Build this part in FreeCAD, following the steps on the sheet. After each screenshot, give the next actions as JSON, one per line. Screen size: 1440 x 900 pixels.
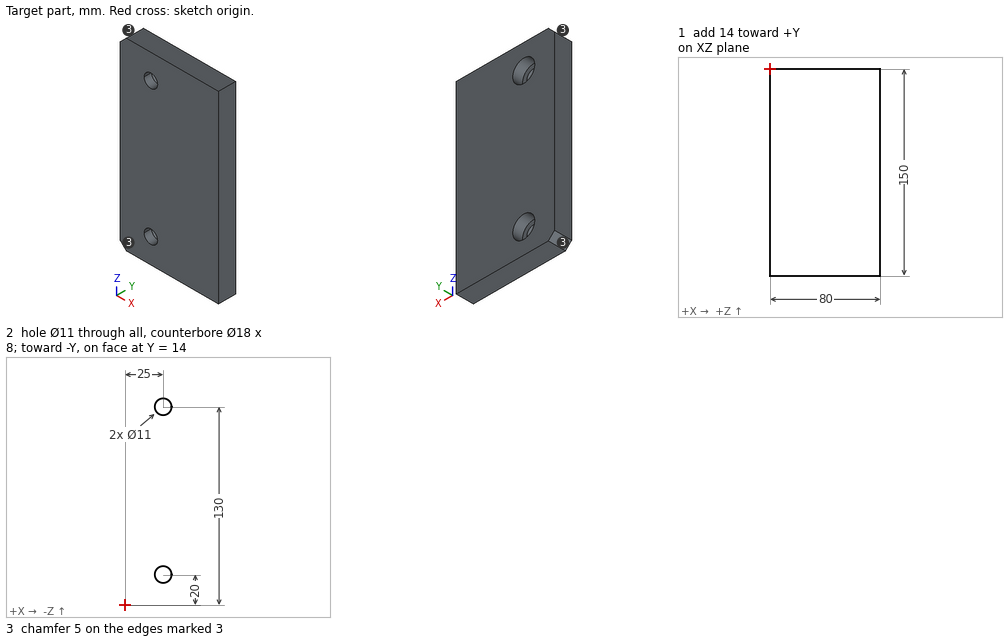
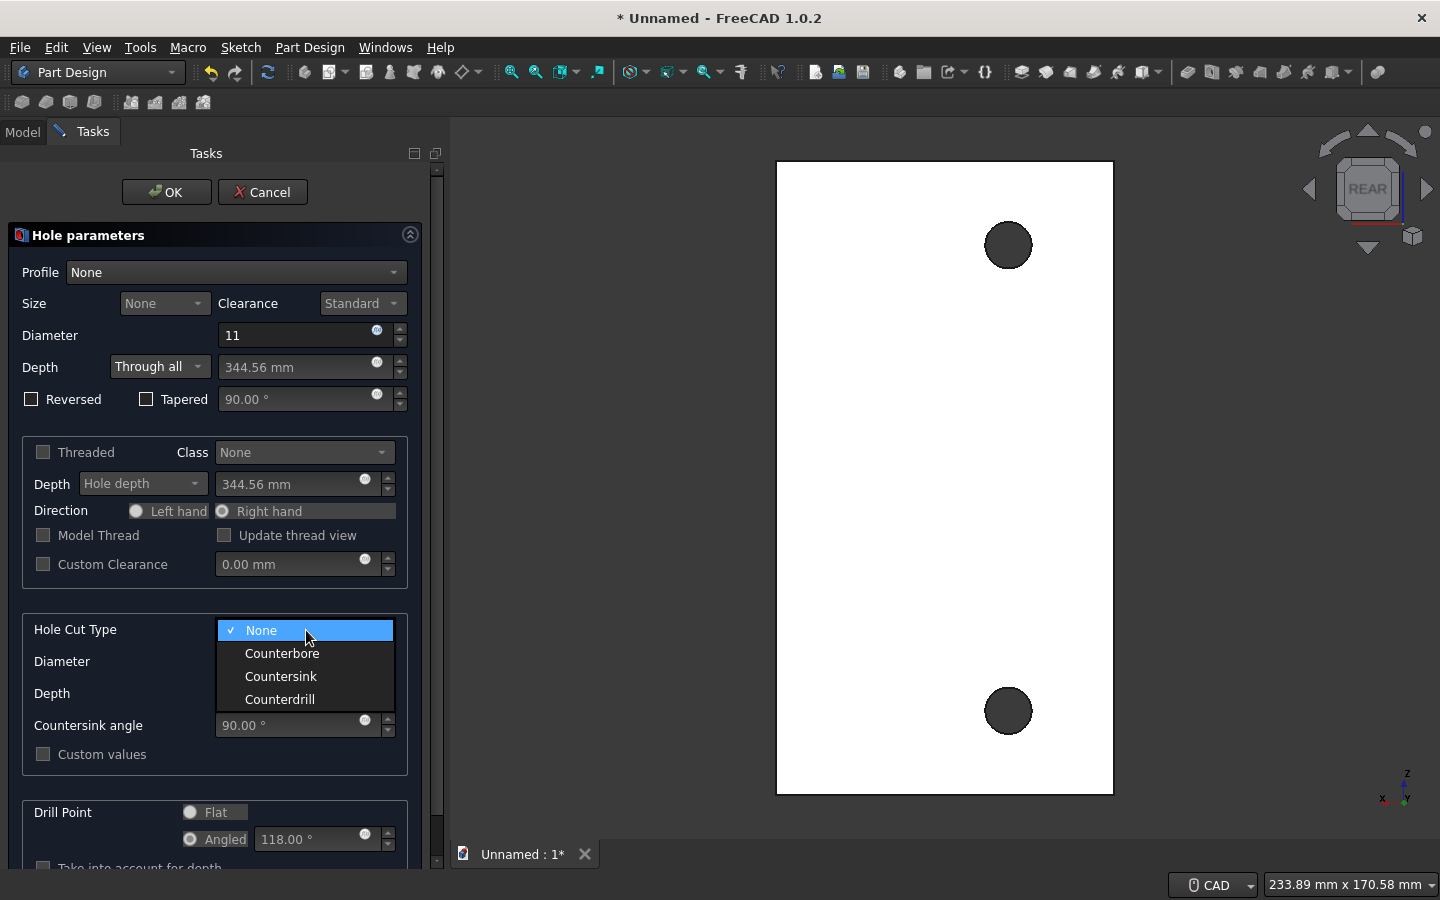
{"action": "left_click", "coordinate": [304, 654]}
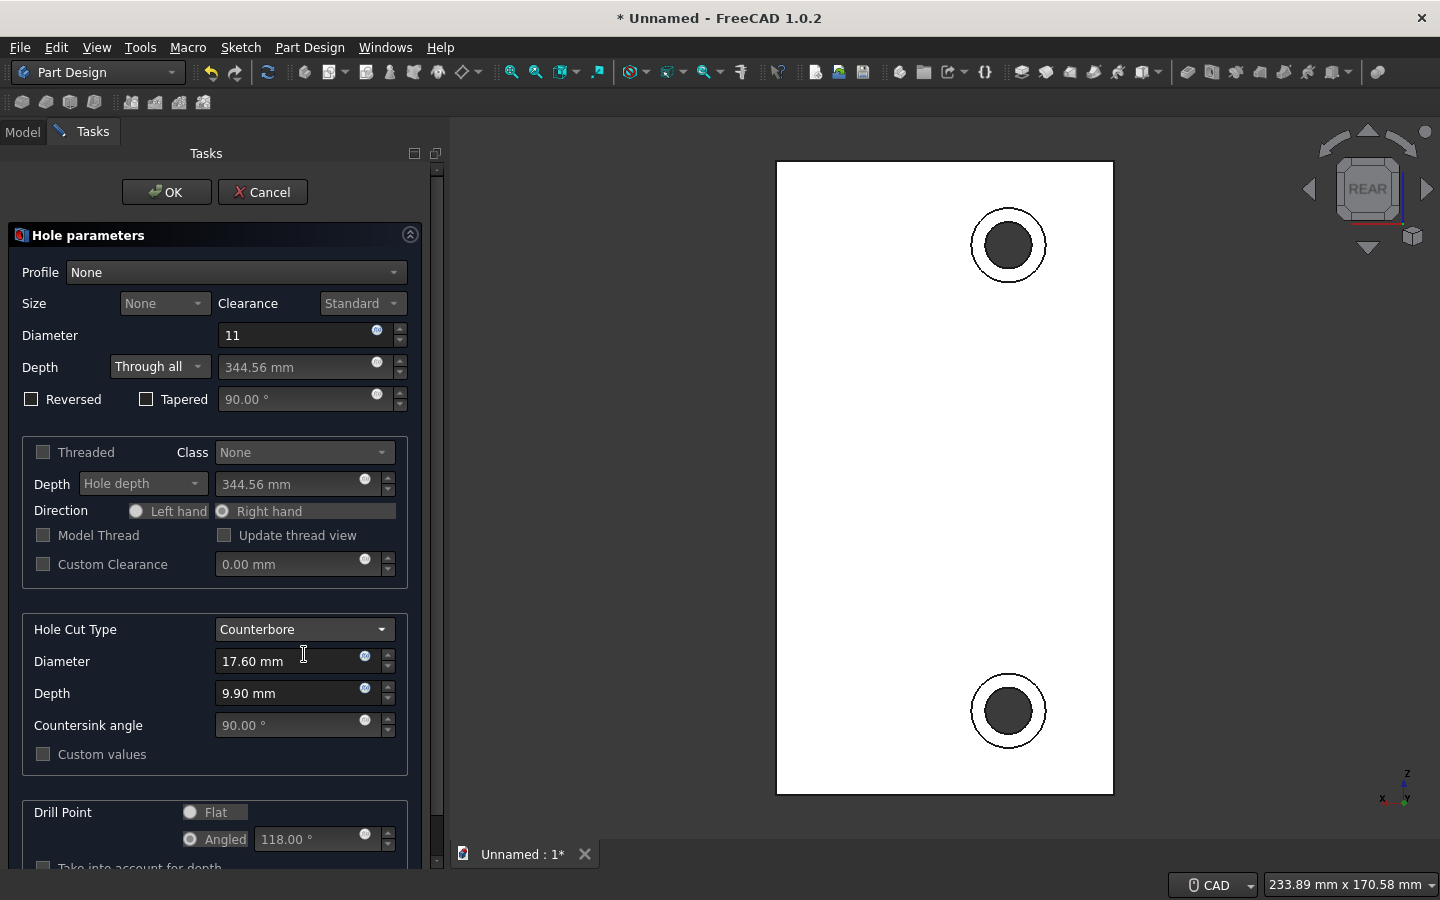
{"action": "triple_click", "coordinate": [298, 661]}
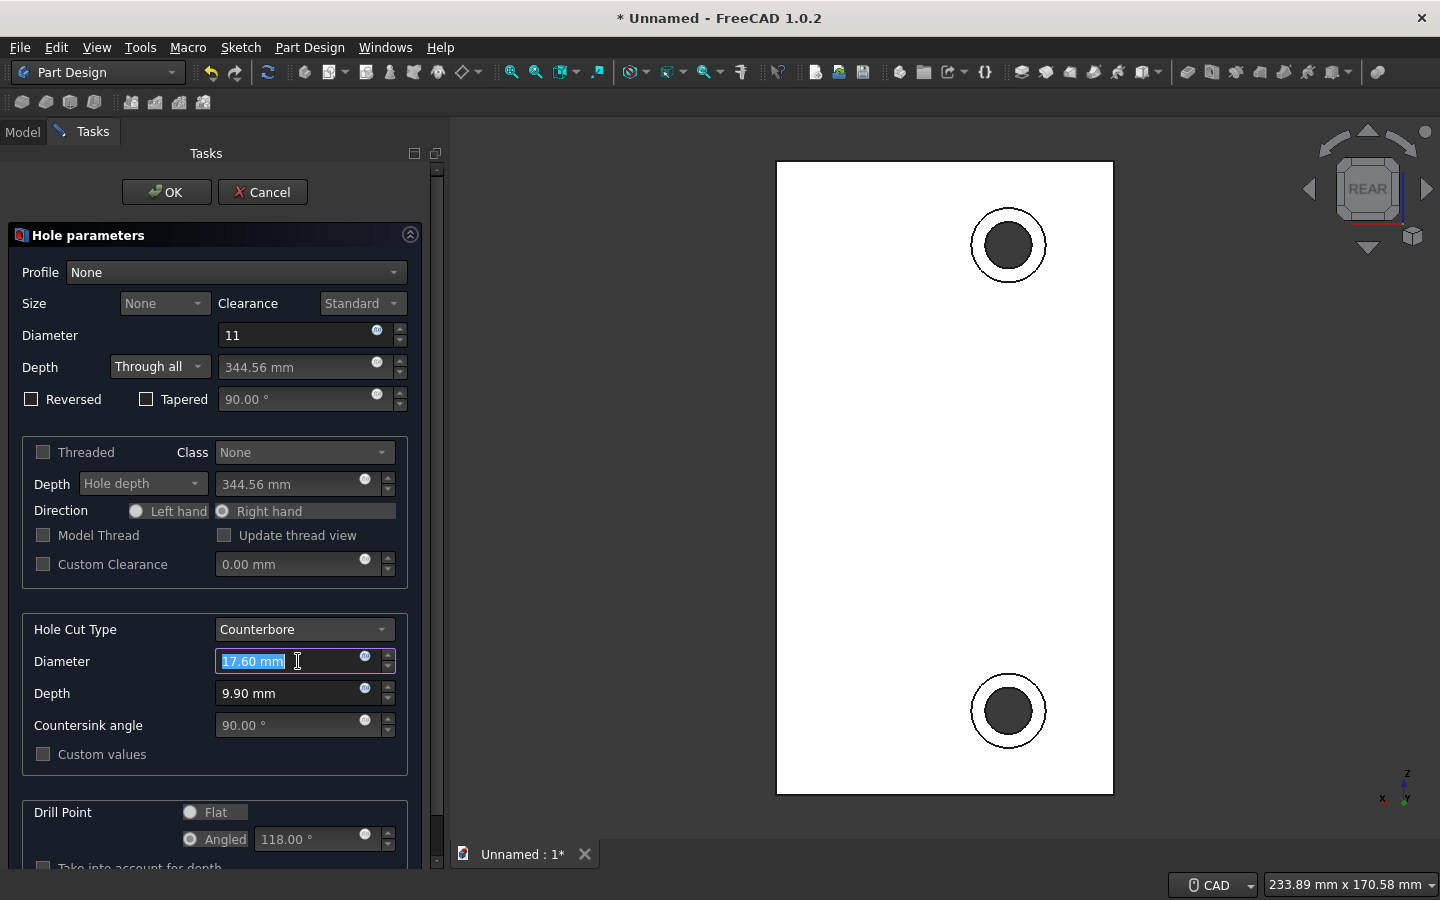
{"action": "type", "text": "18"}
{"action": "key", "text": "Tab"}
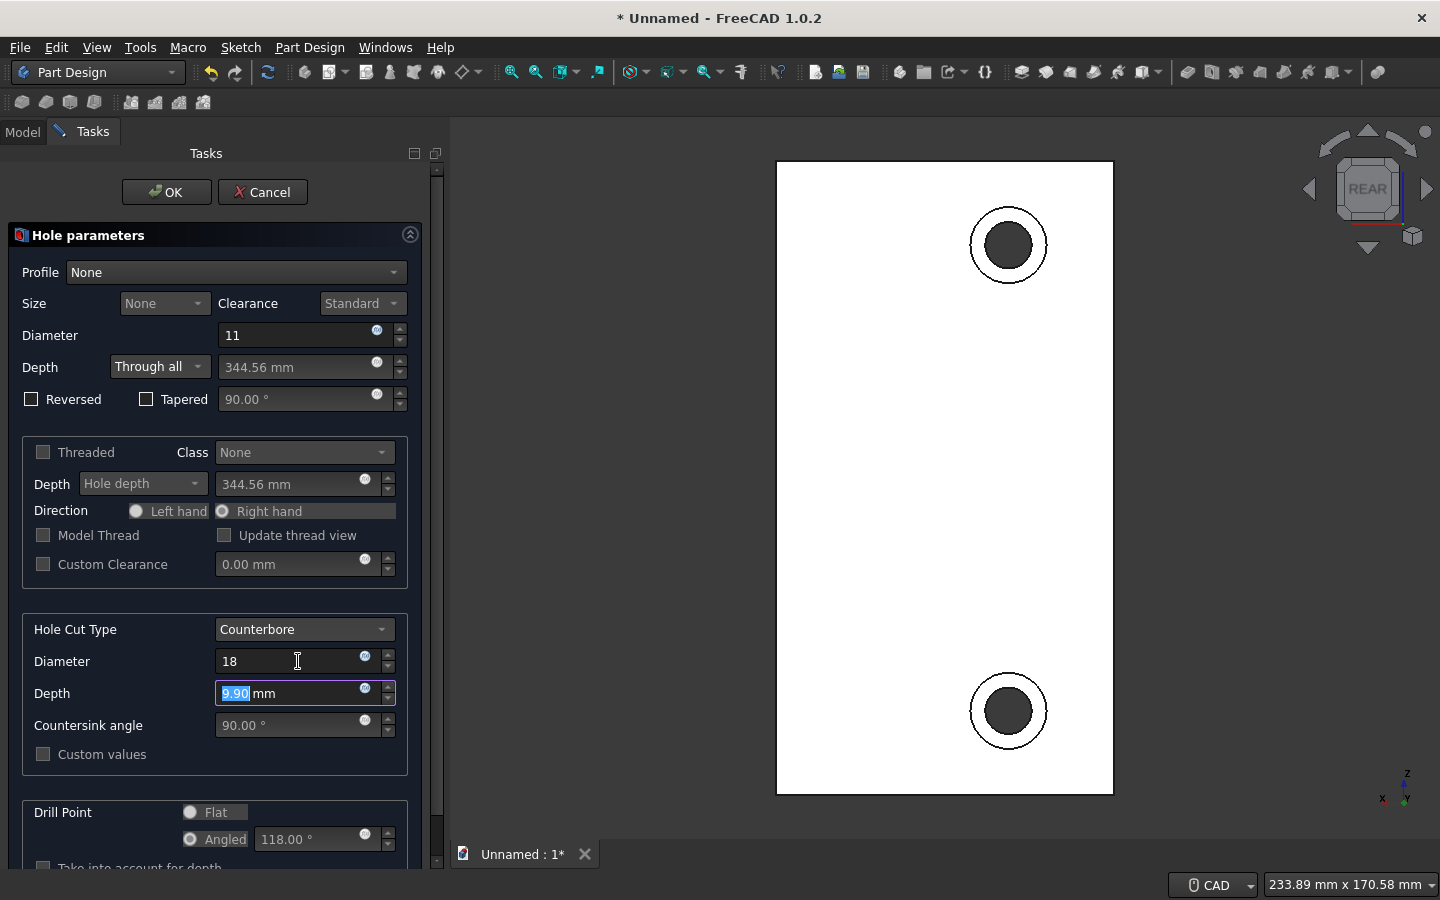
{"action": "type", "text": "8"}
{"action": "key", "text": "Tab"}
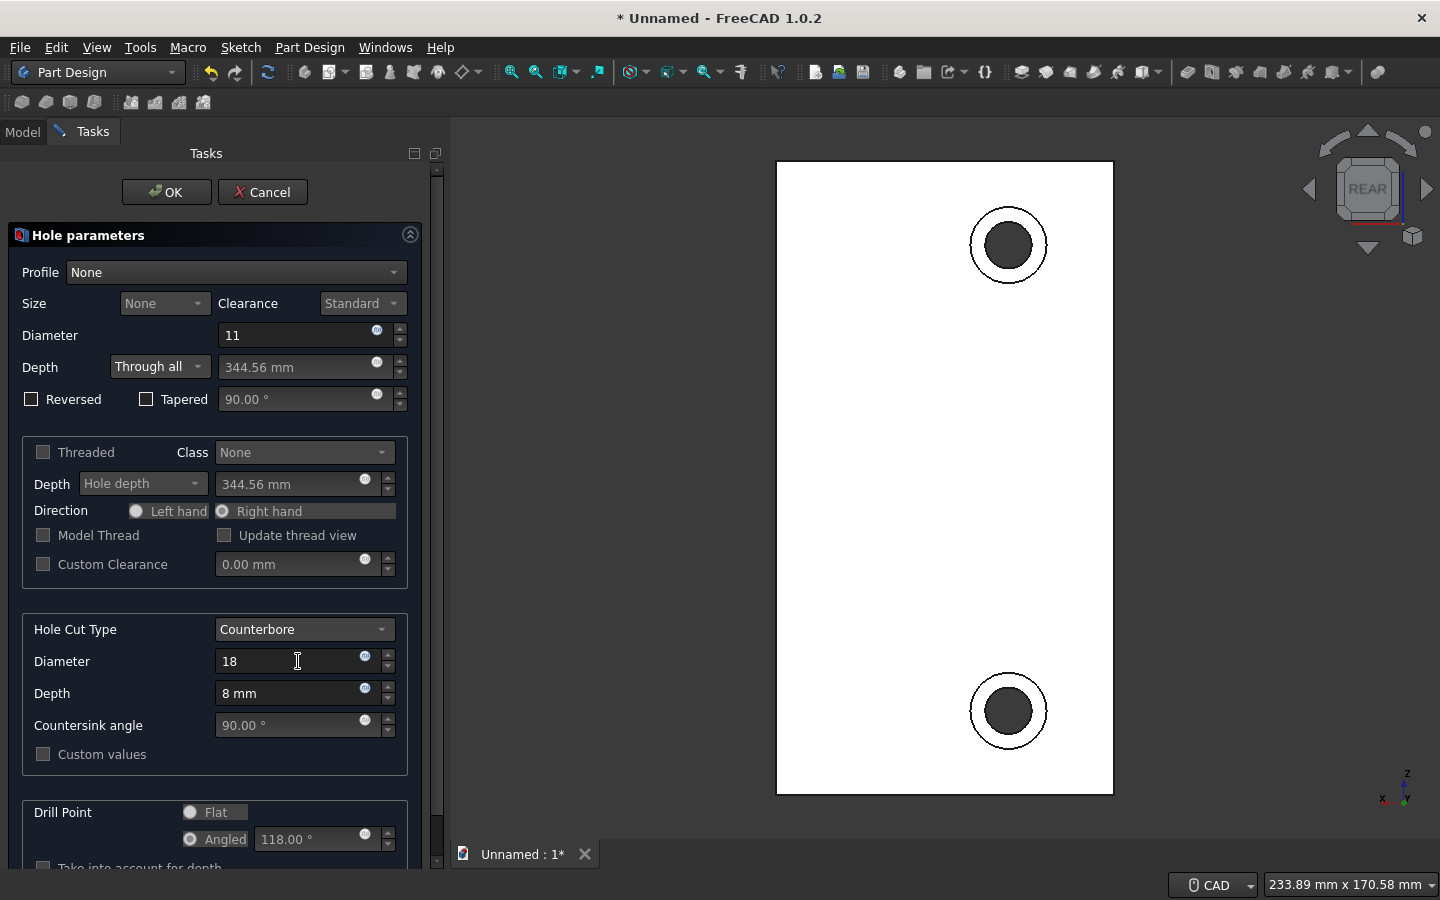
{"action": "left_click", "coordinate": [167, 192]}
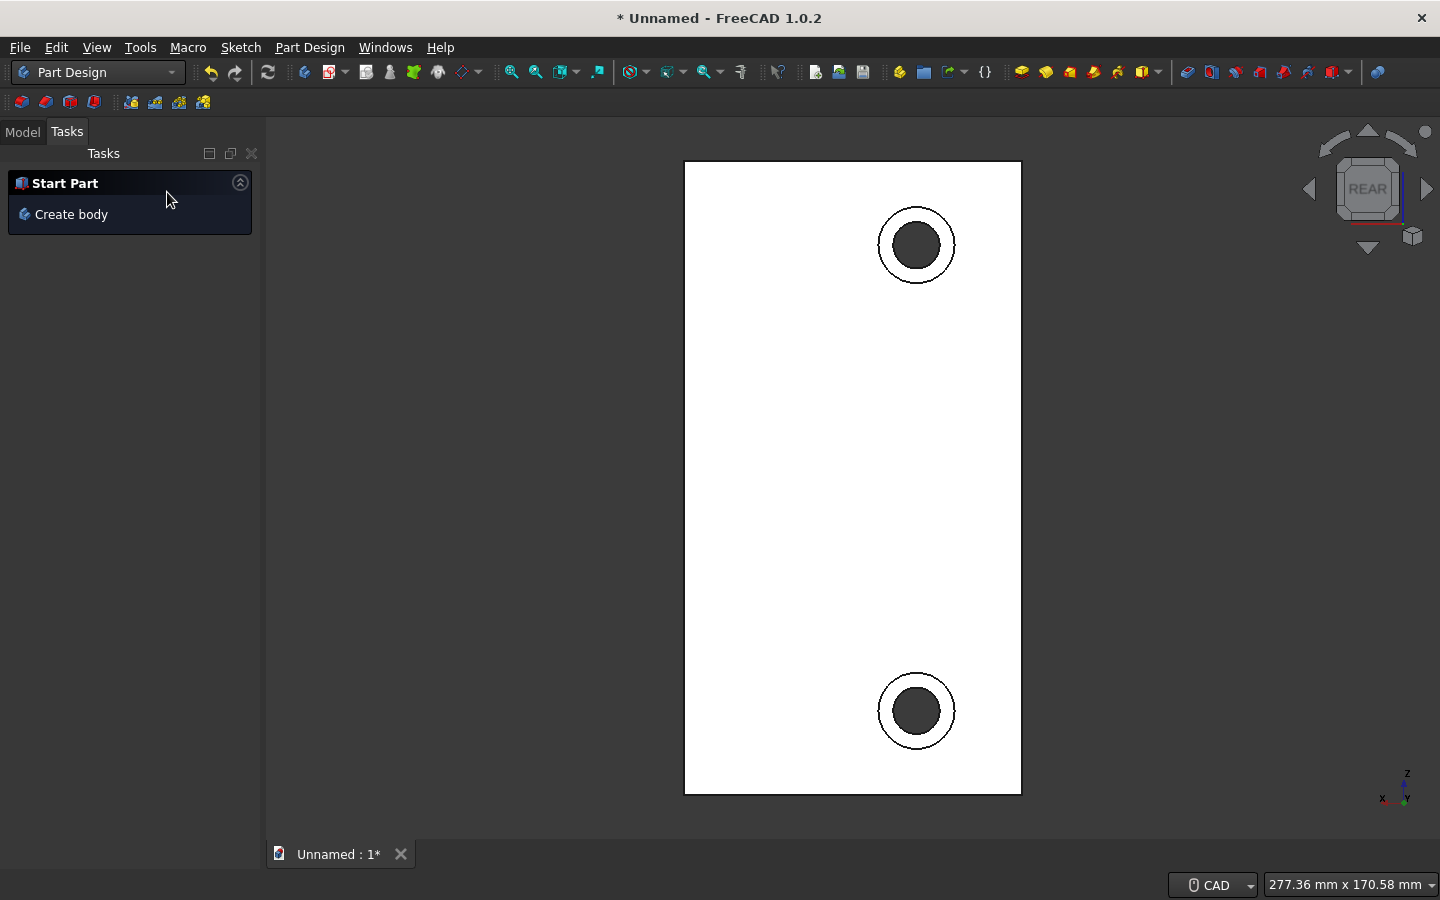
{"action": "key", "text": "0"}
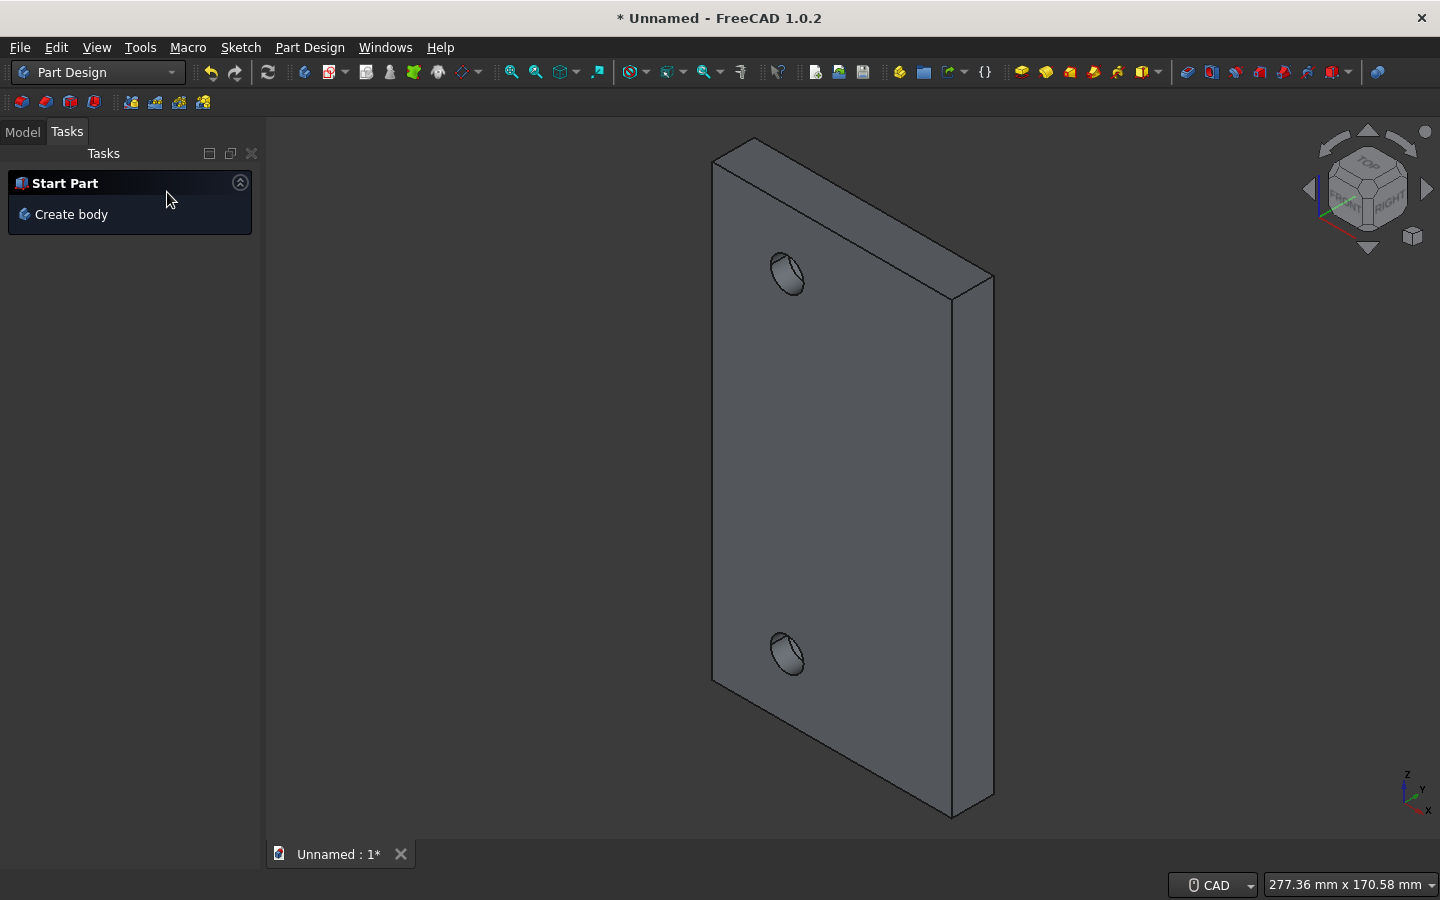
{"action": "key", "text": "2"}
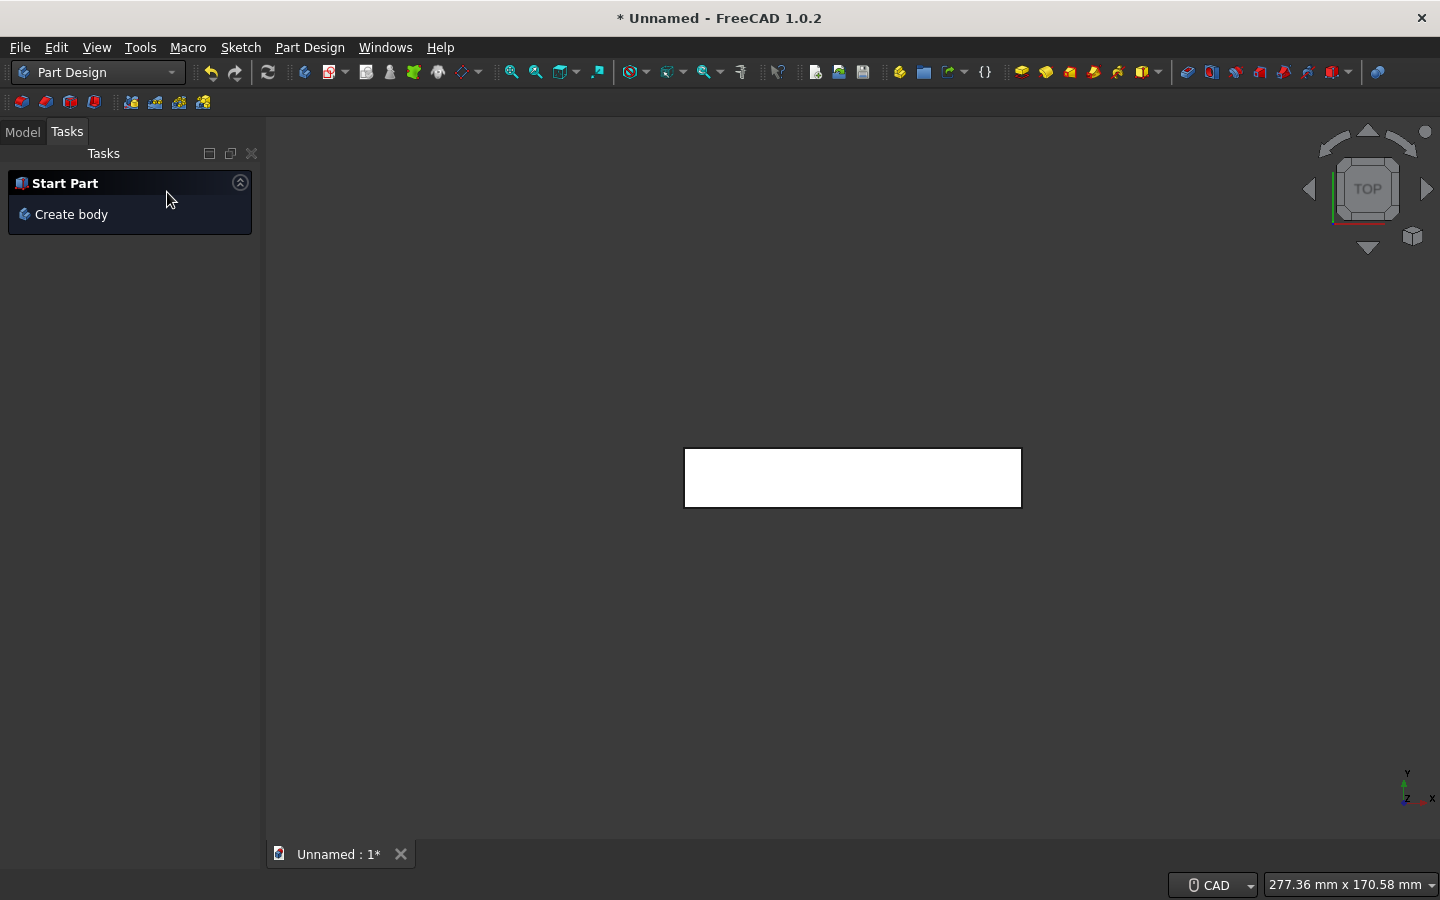
{"action": "left_click", "coordinate": [512, 72]}